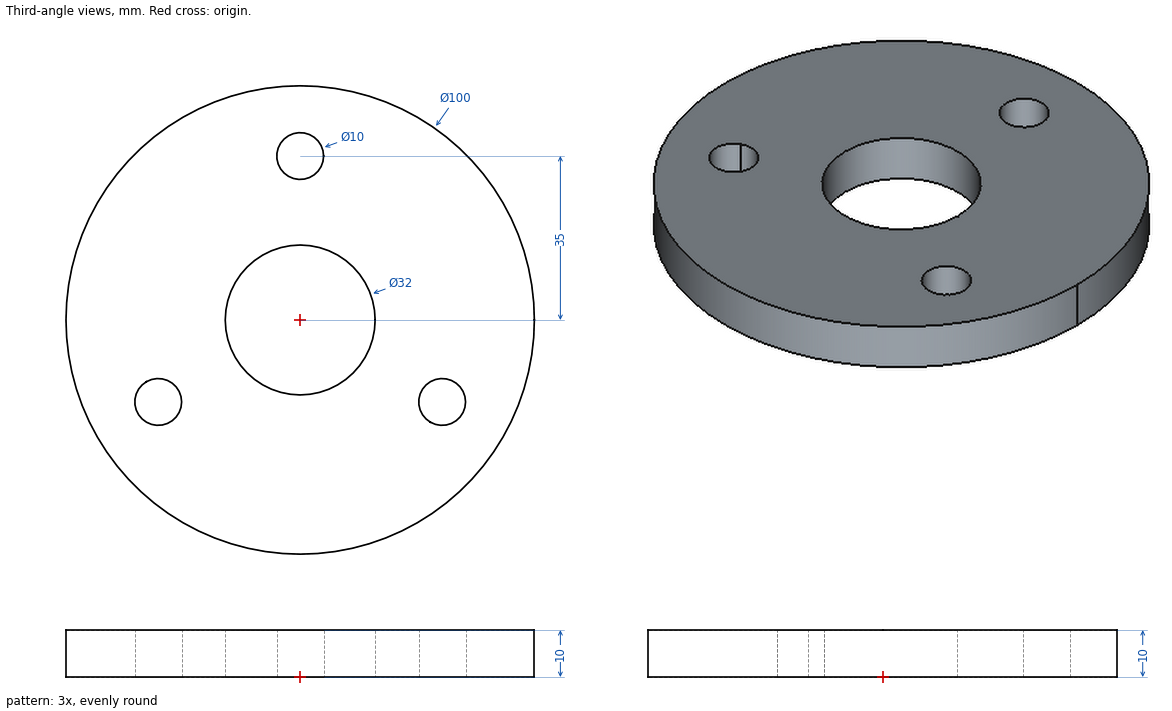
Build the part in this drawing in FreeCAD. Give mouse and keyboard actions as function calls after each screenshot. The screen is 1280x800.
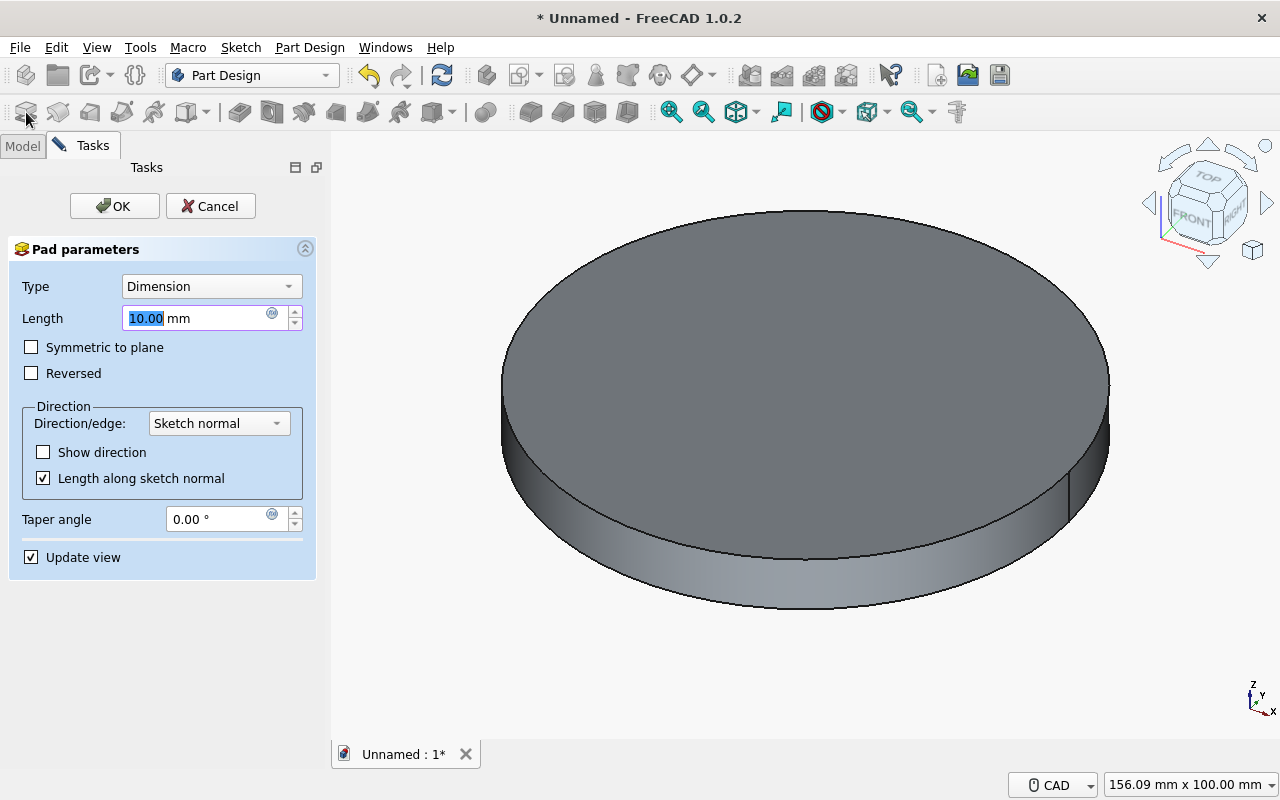
text(10)
key(Tab)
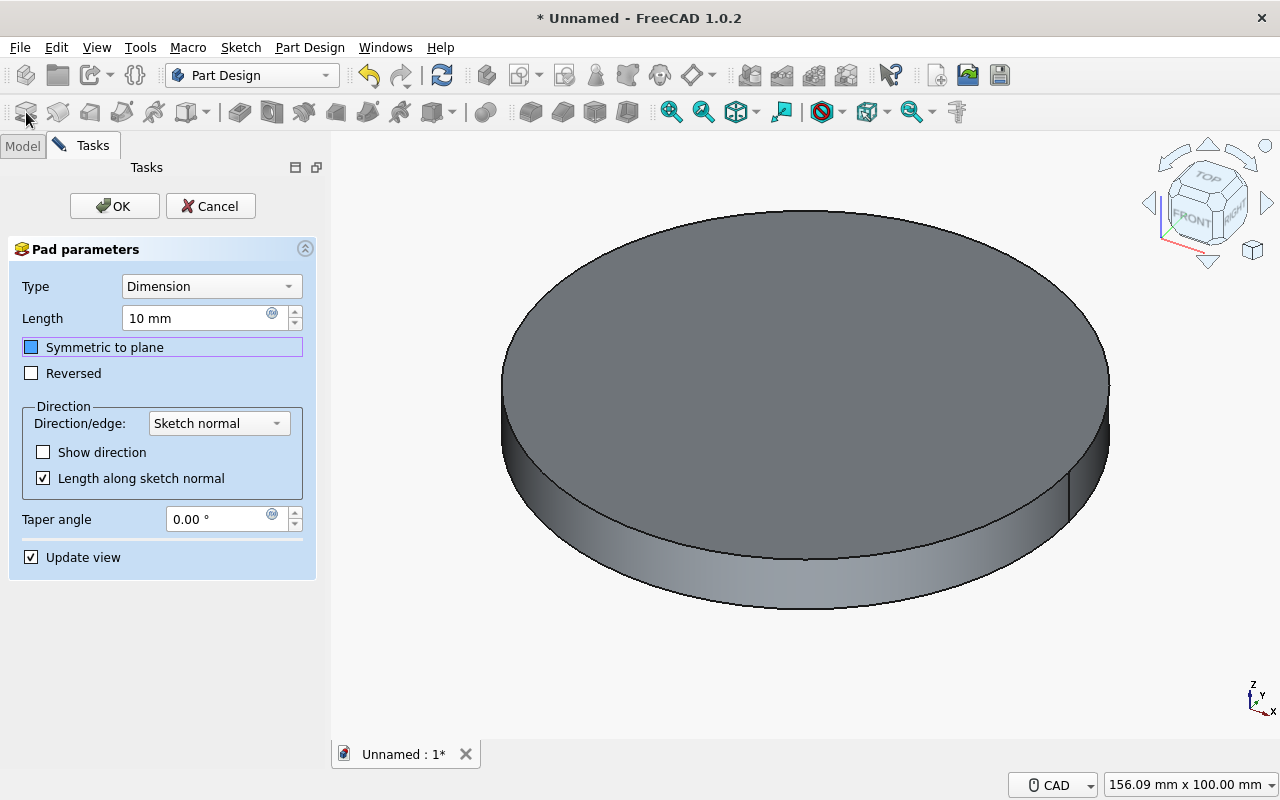
click(115, 206)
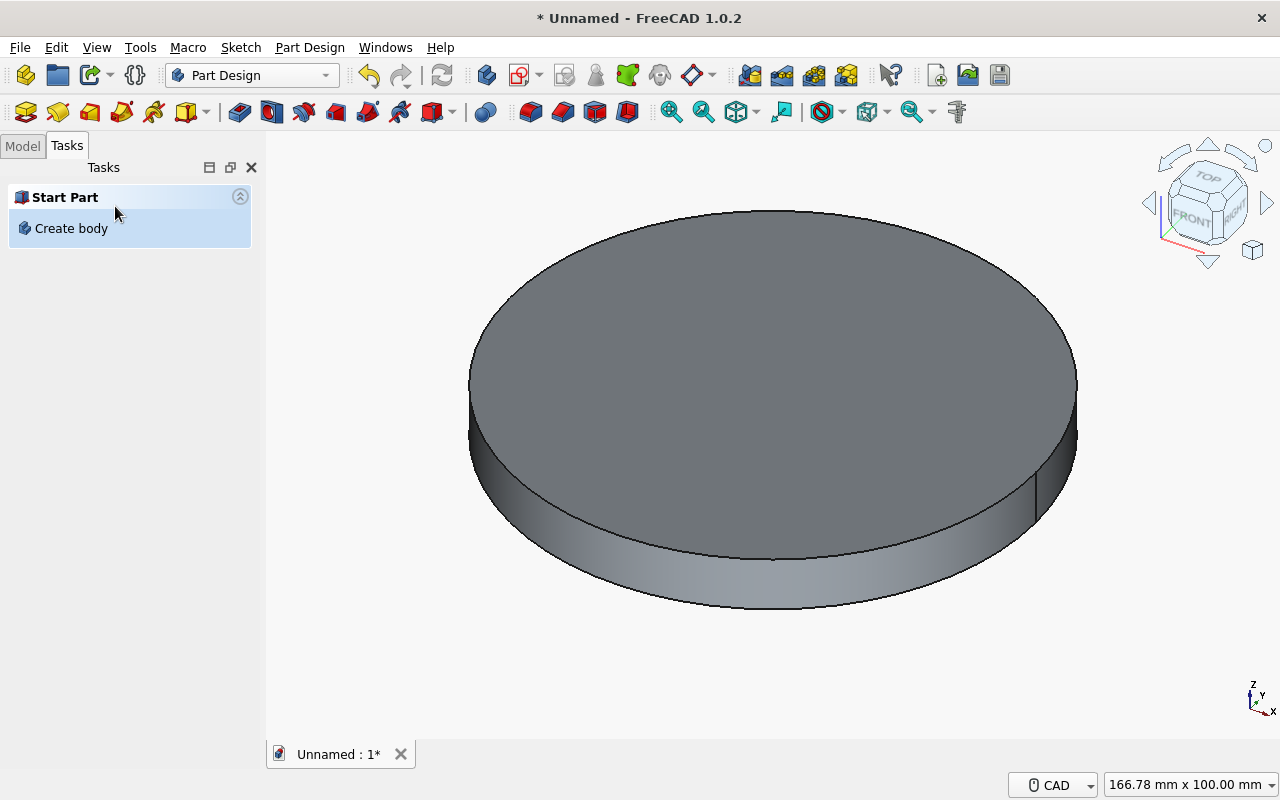
click(773, 384)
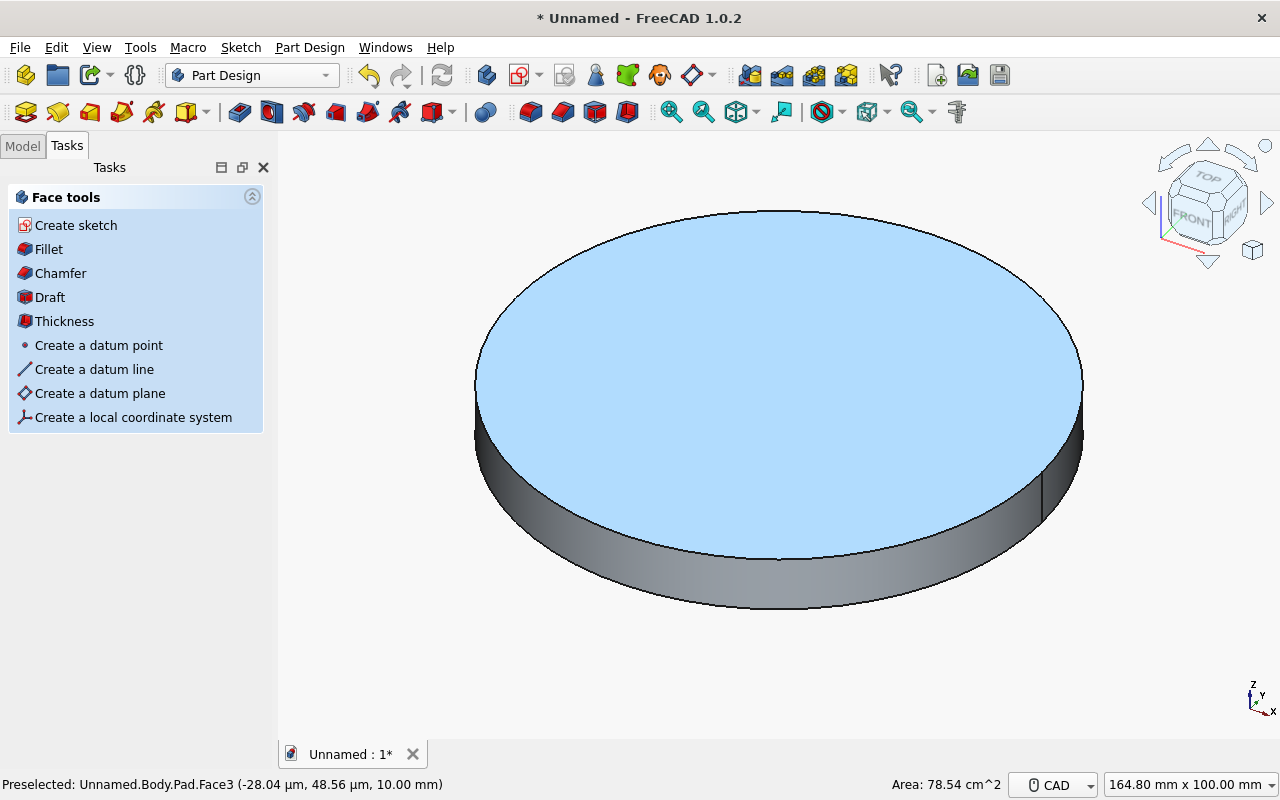
click(520, 76)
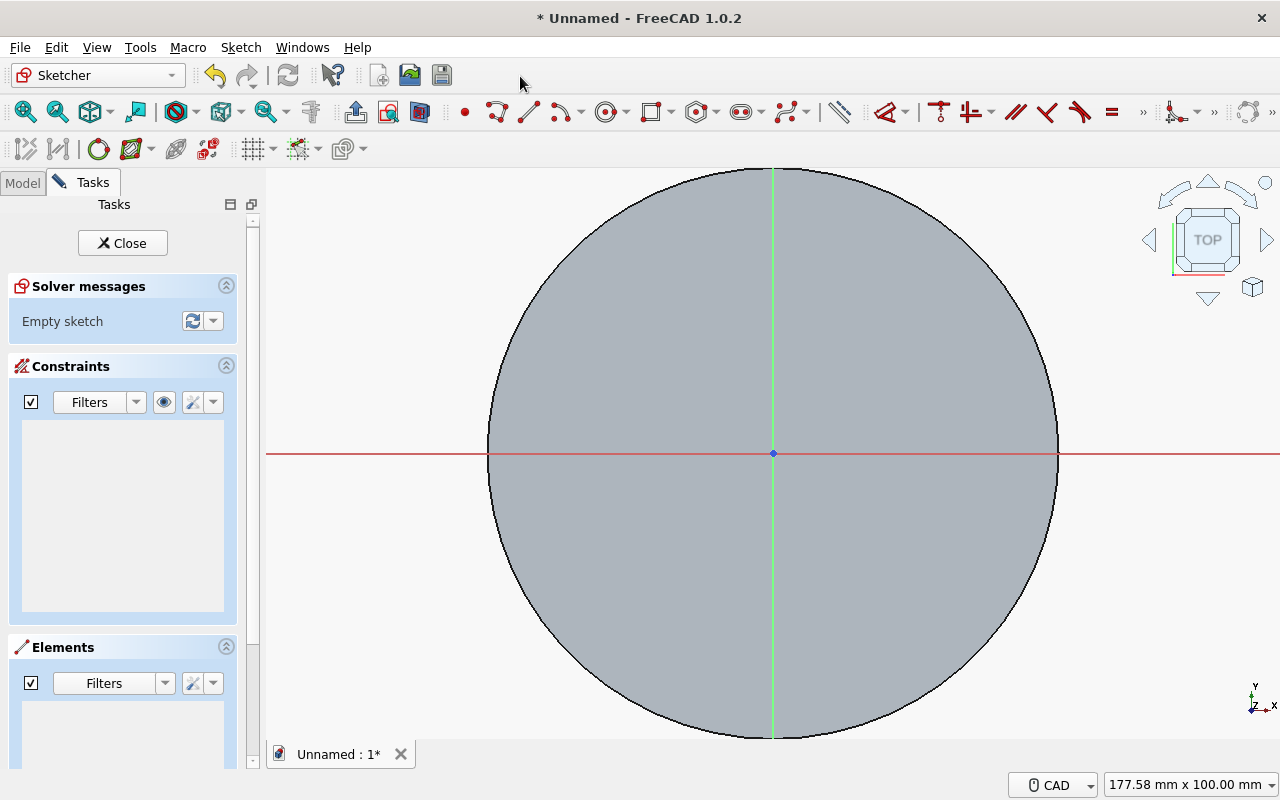
scroll(787, 214, up, 9)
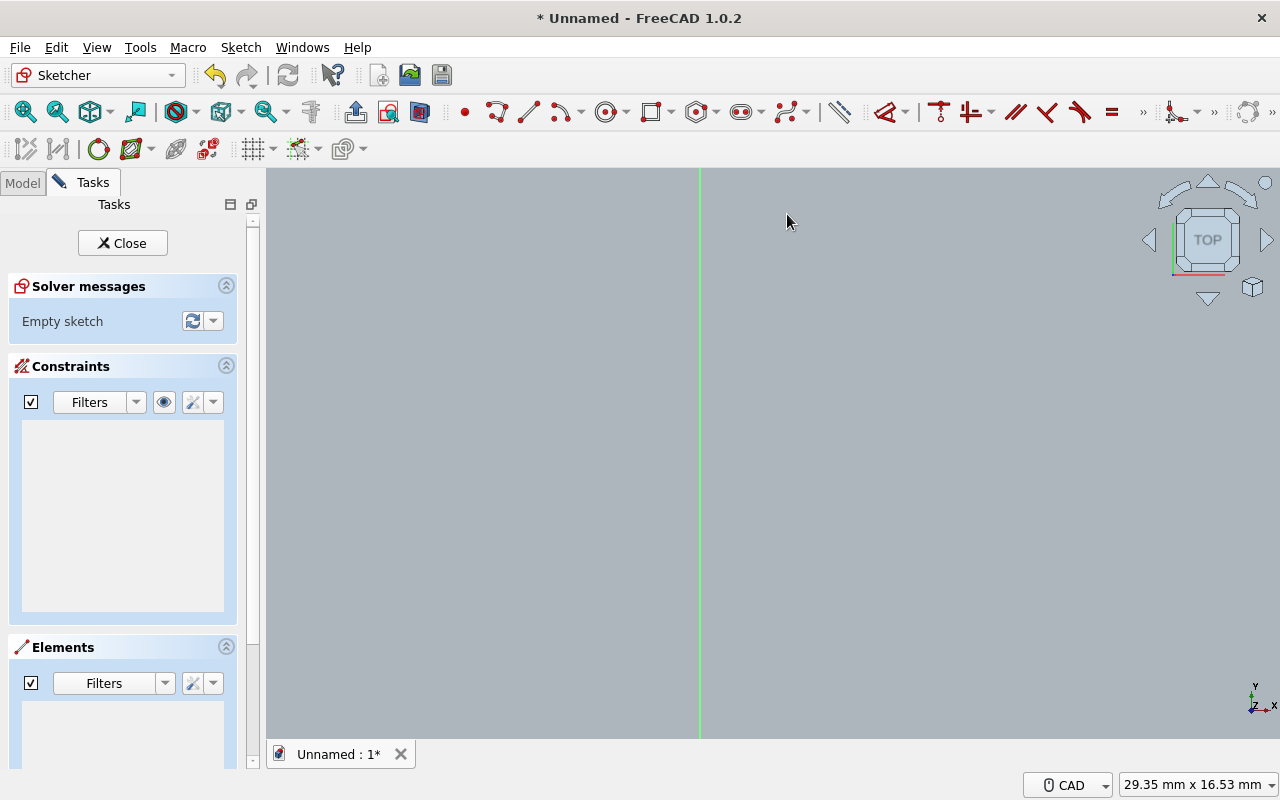
click(606, 112)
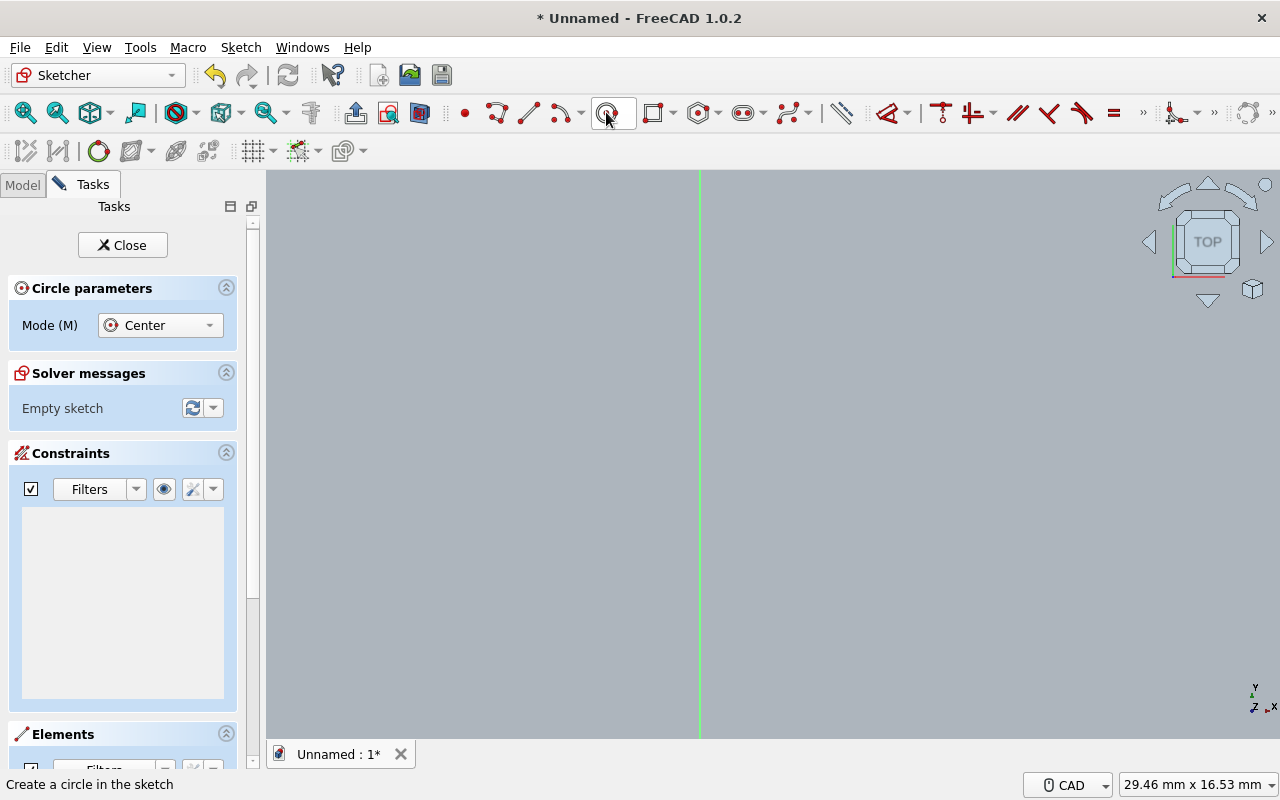
click(700, 454)
move(822, 333)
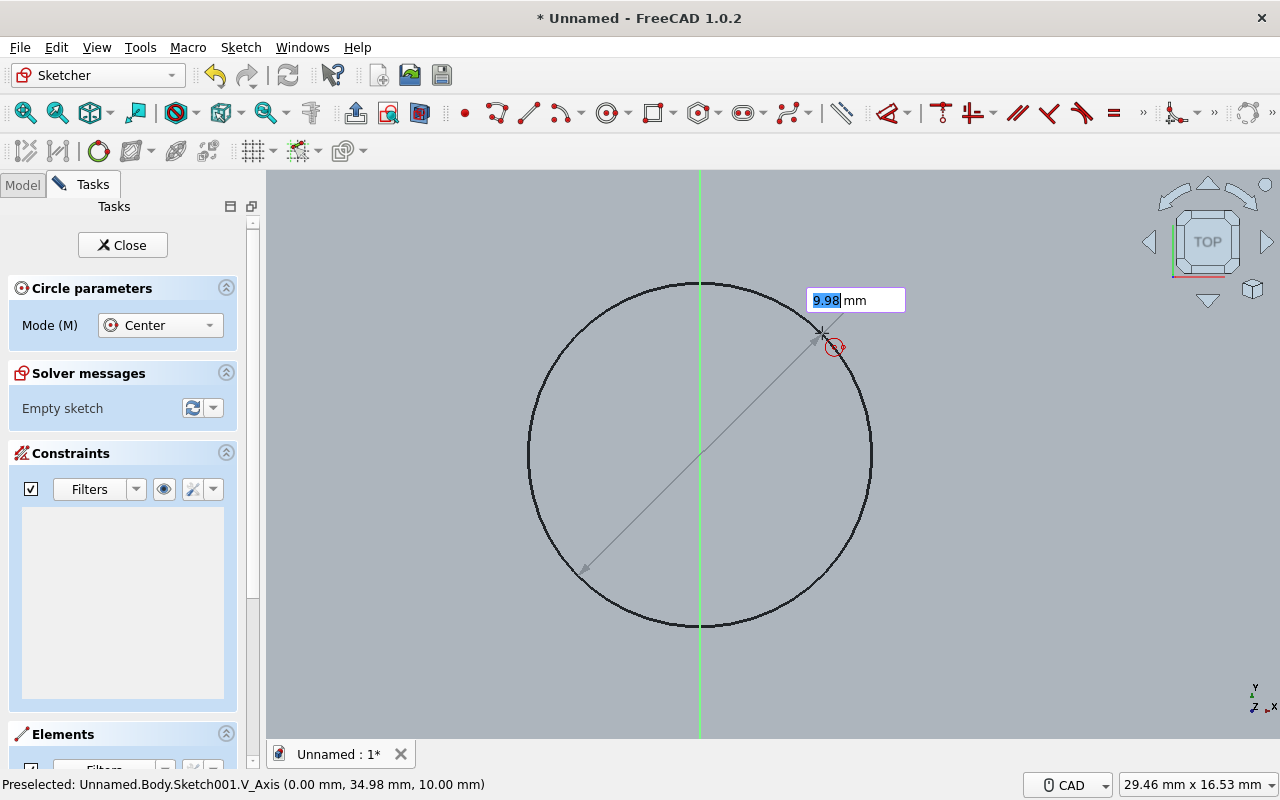
text(10)
key(Return)
key(Escape)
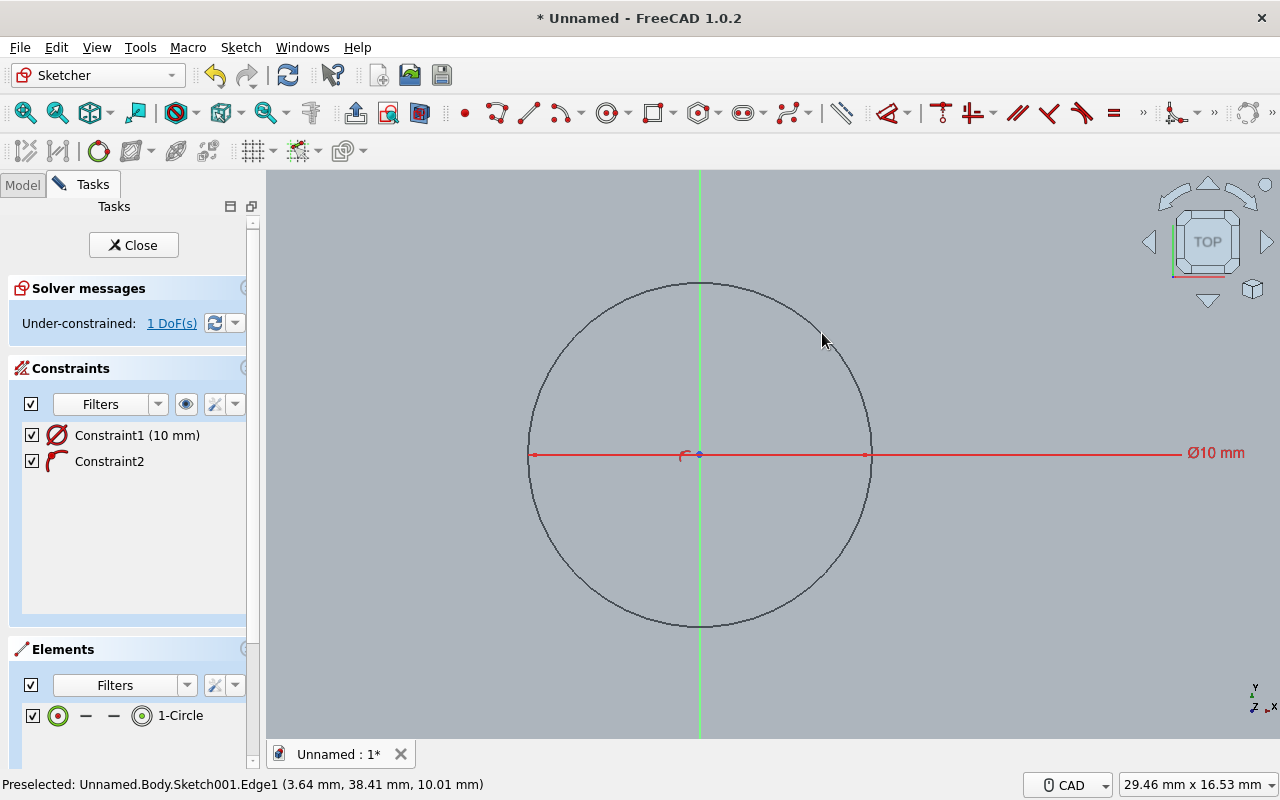
click(888, 114)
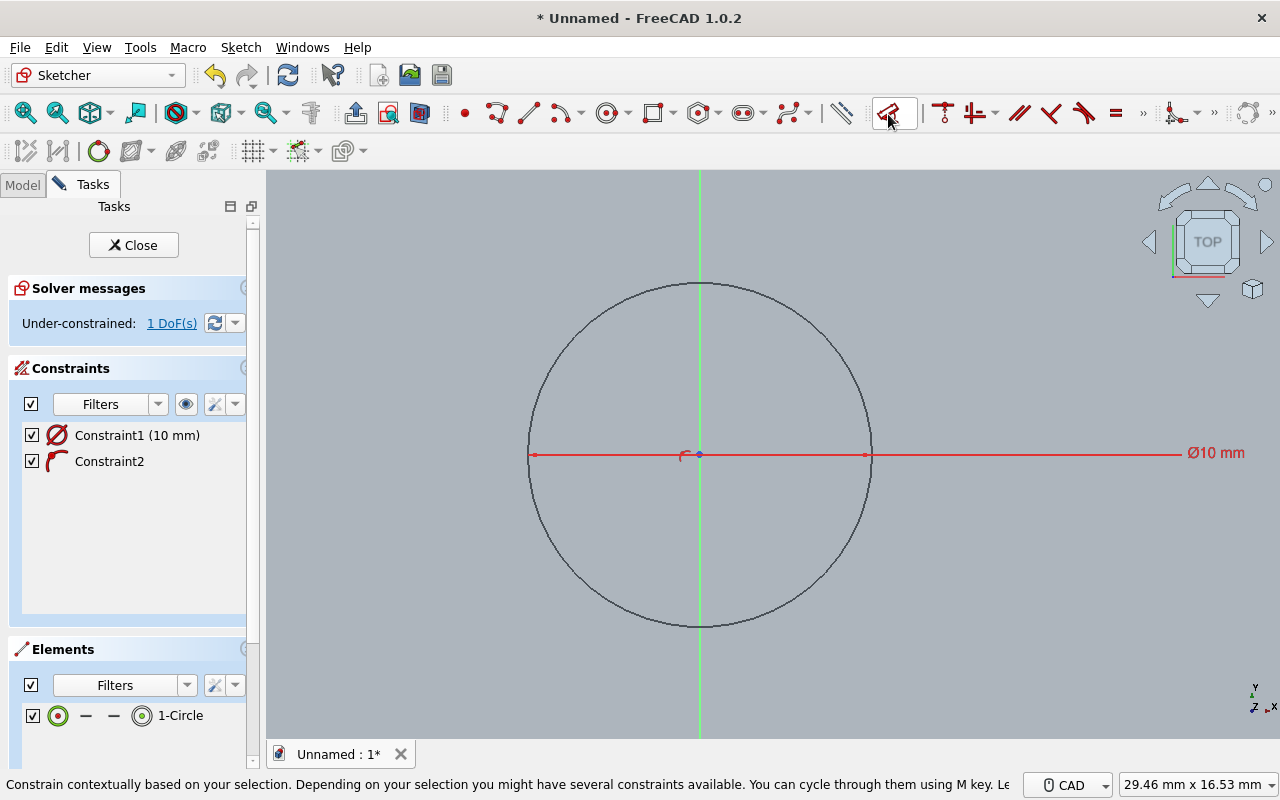
click(700, 455)
click(734, 583)